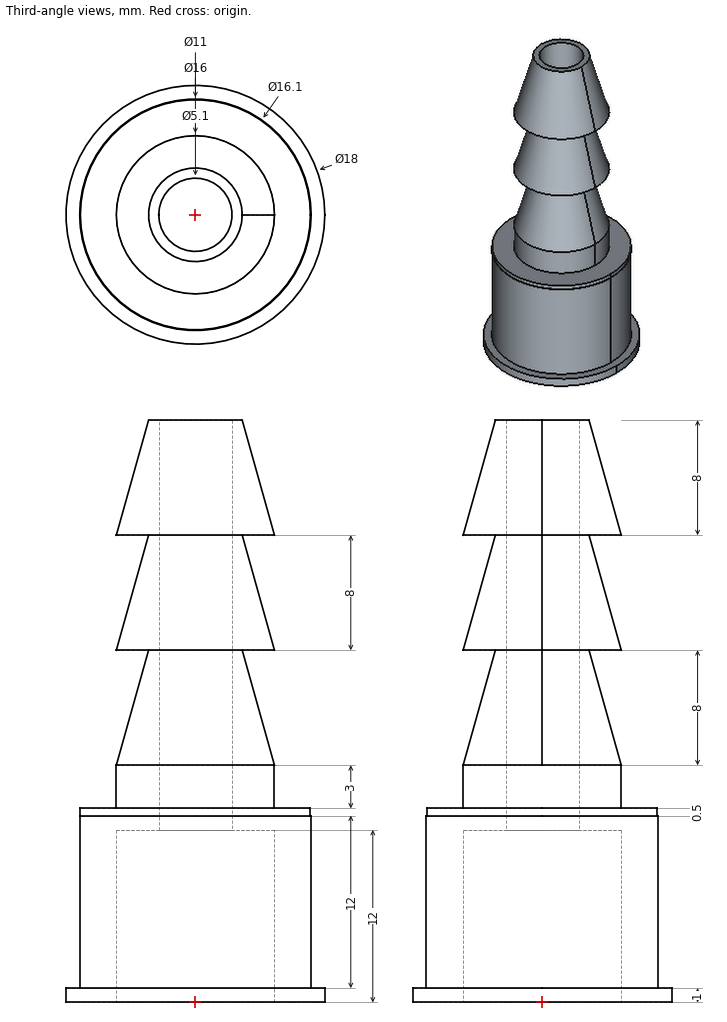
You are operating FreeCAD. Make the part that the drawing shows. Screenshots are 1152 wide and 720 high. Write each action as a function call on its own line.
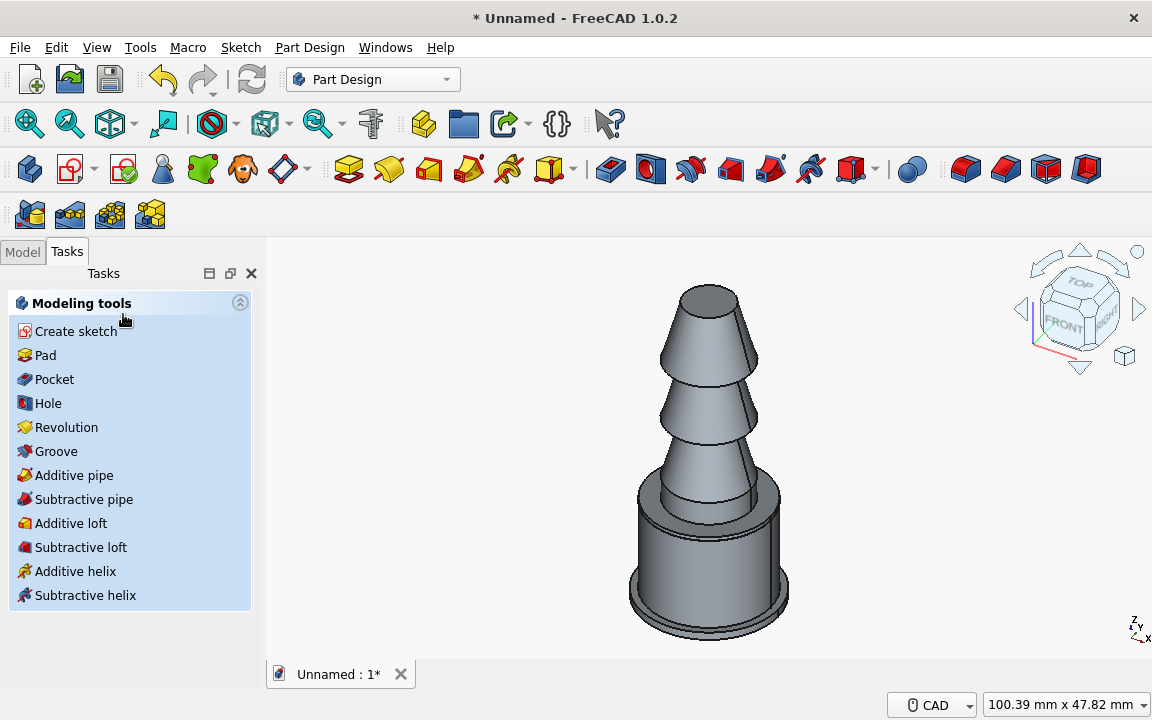
click(612, 170)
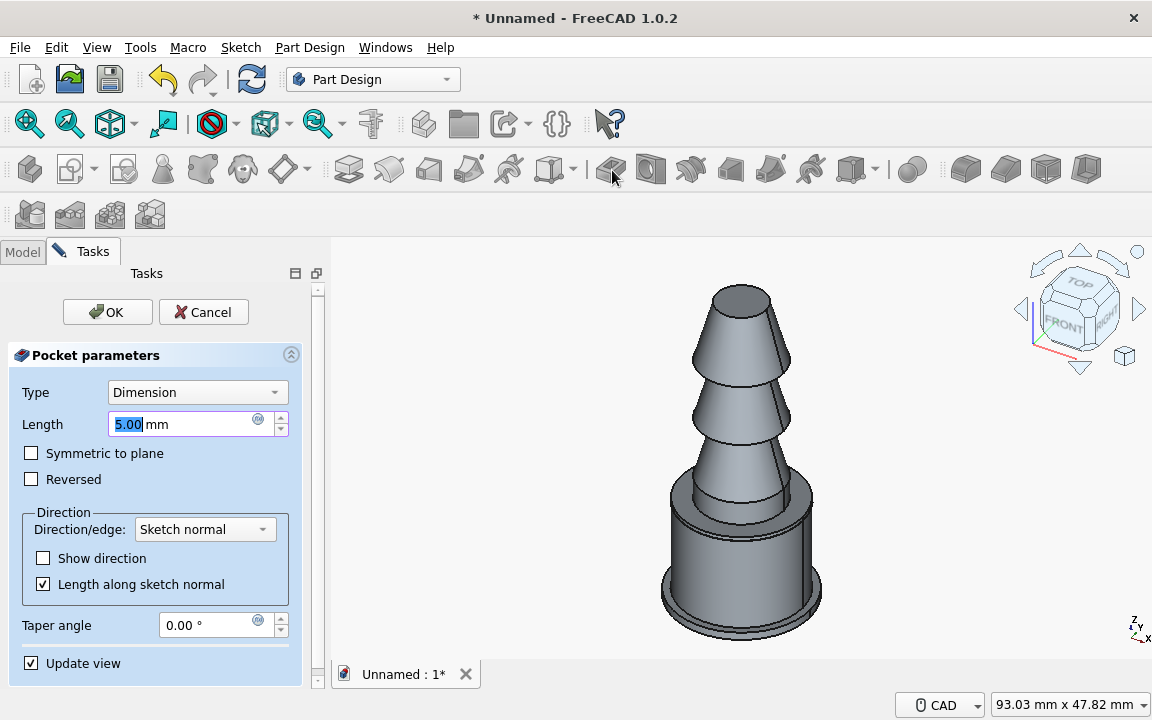
text(12)
key(Tab)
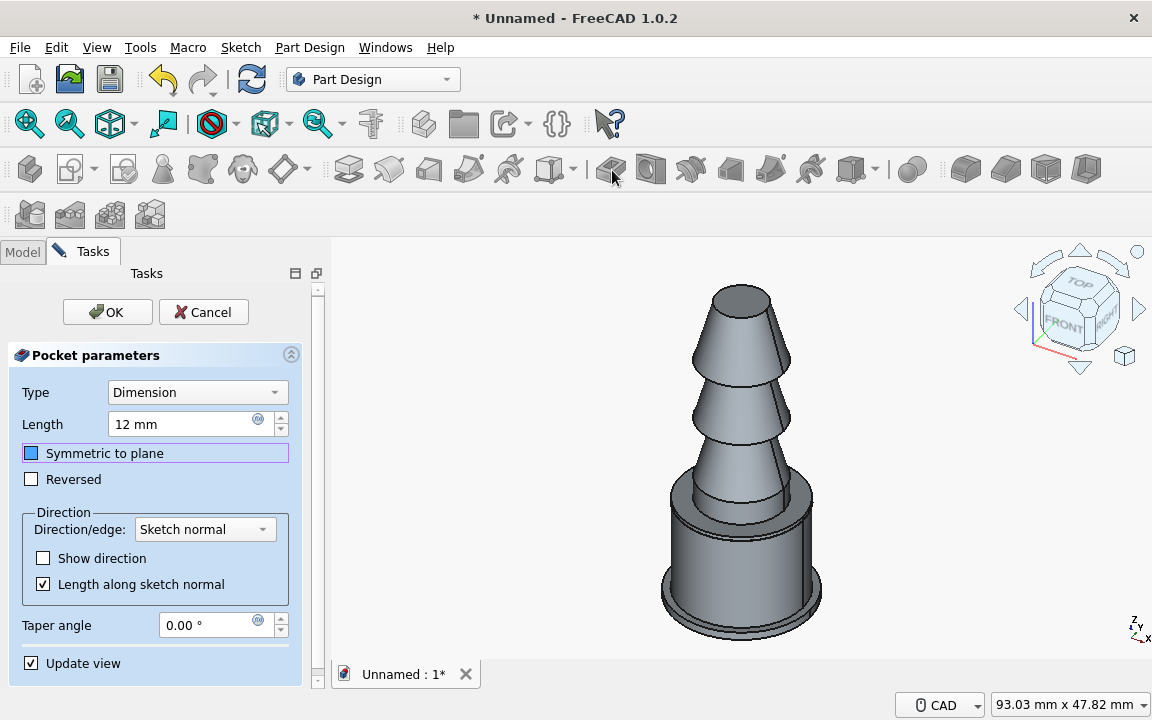
click(30, 479)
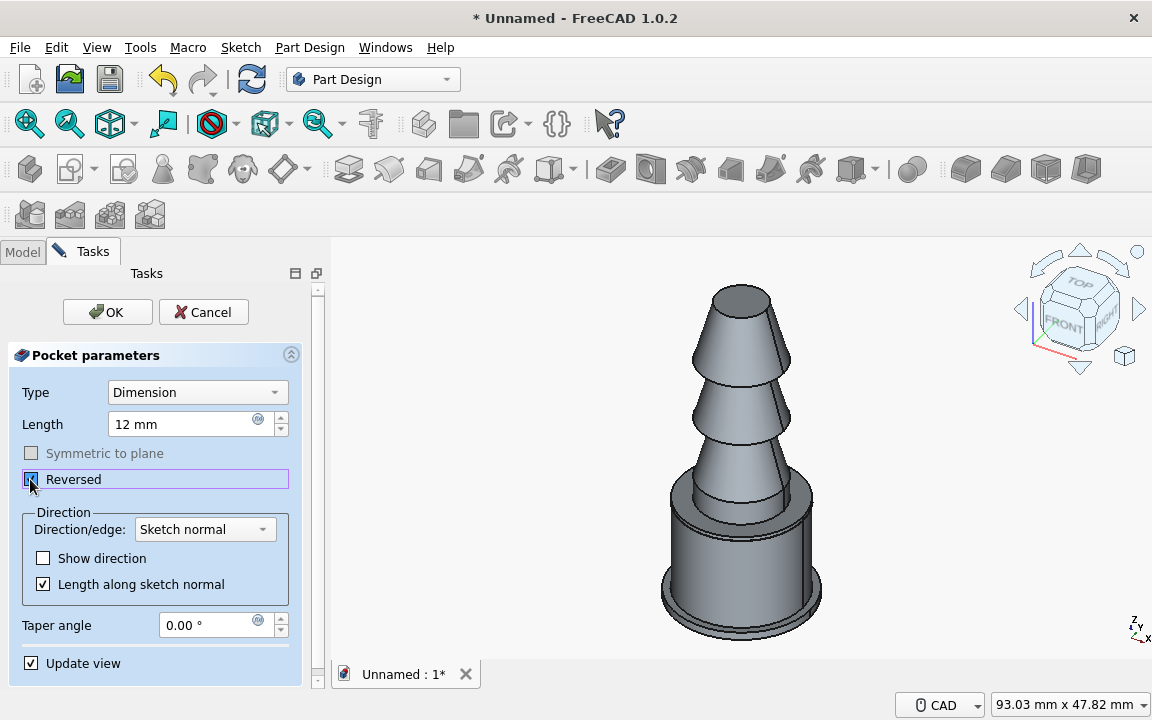
click(108, 312)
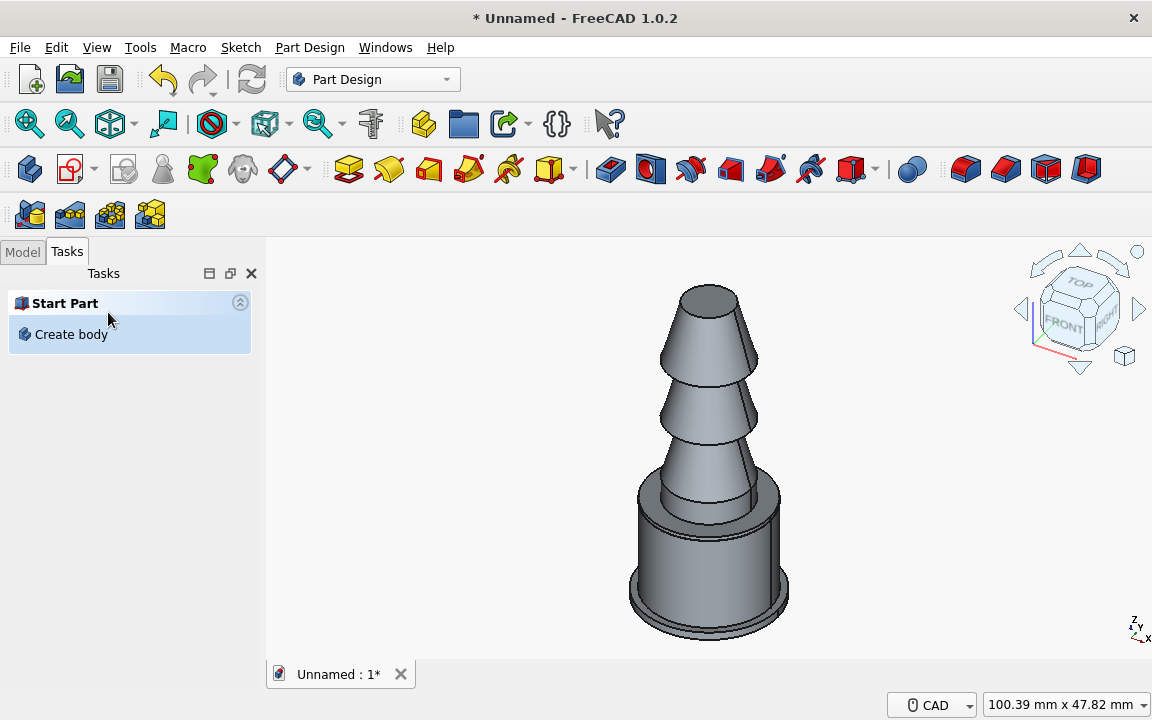
key(5)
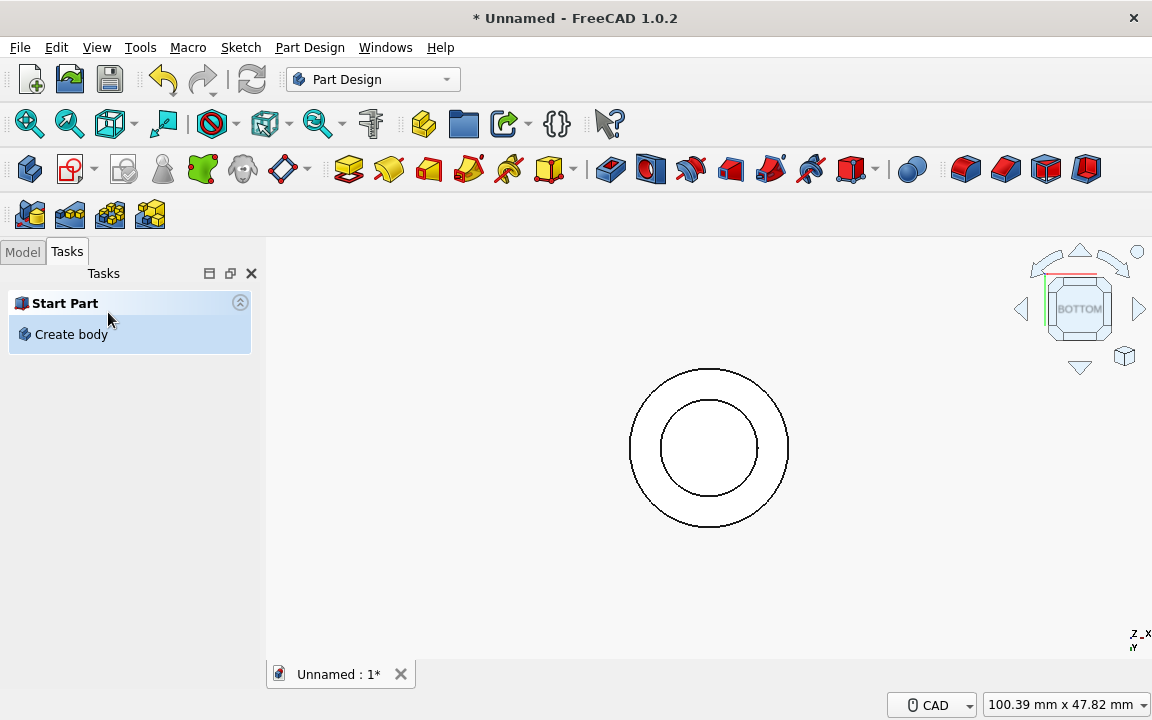
click(30, 124)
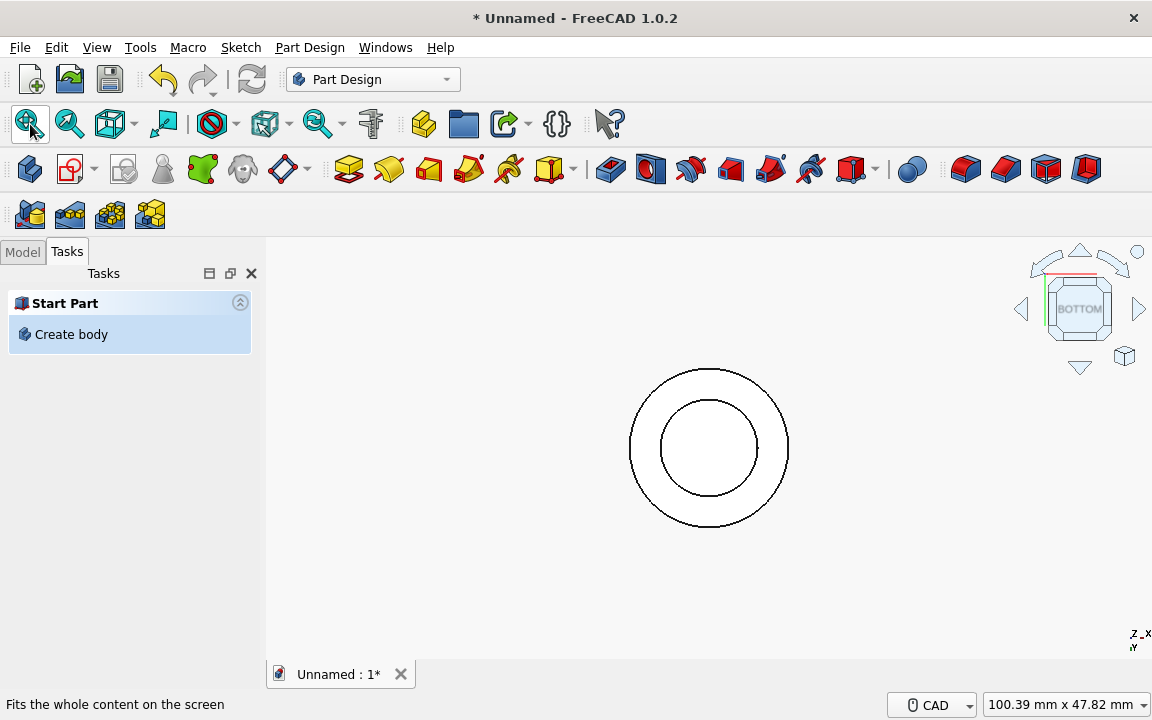
click(709, 447)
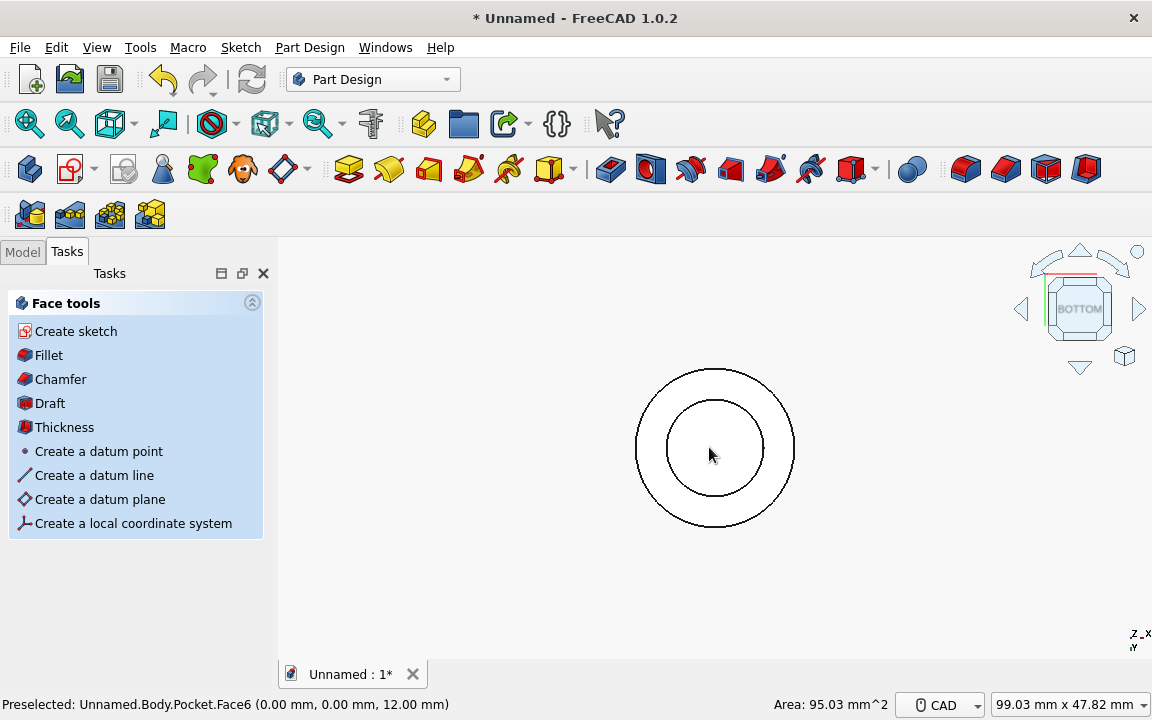
click(70, 170)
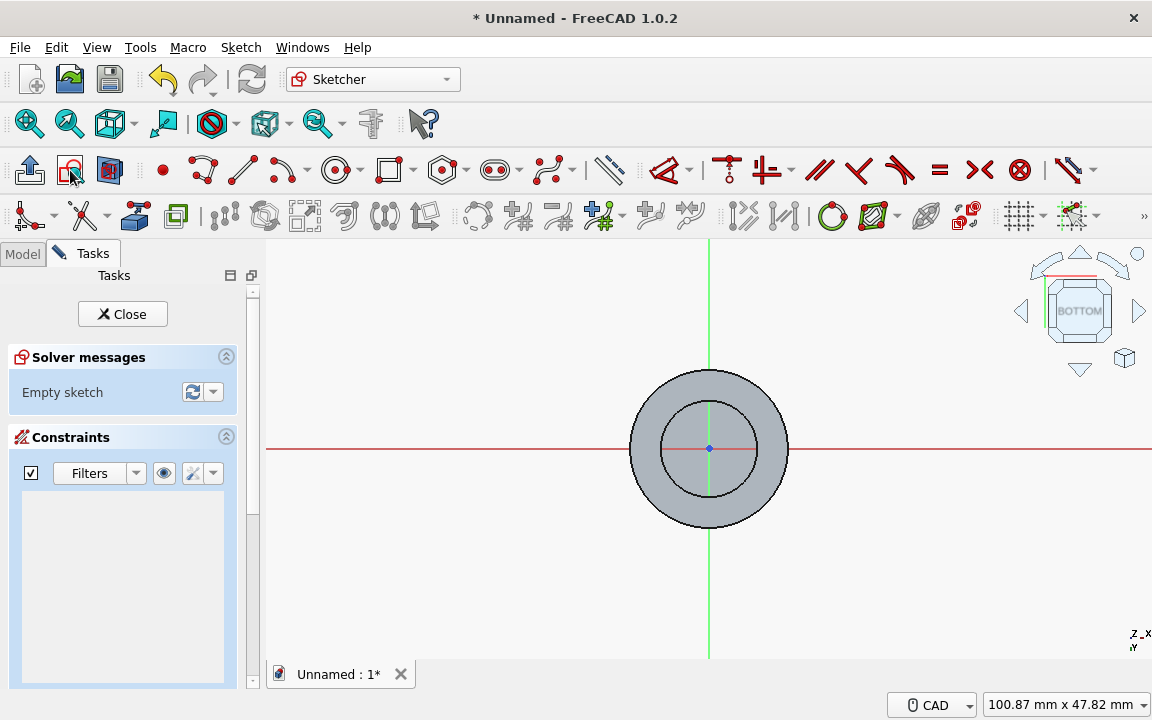
scroll(723, 449, up, 9)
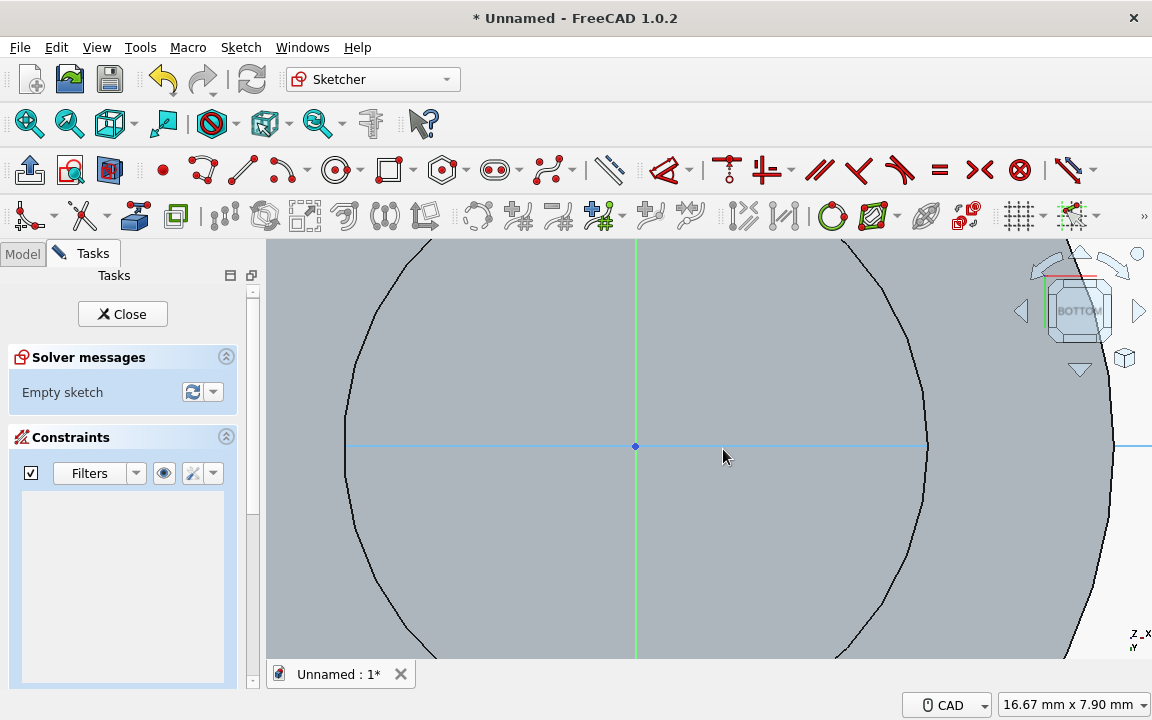
click(336, 170)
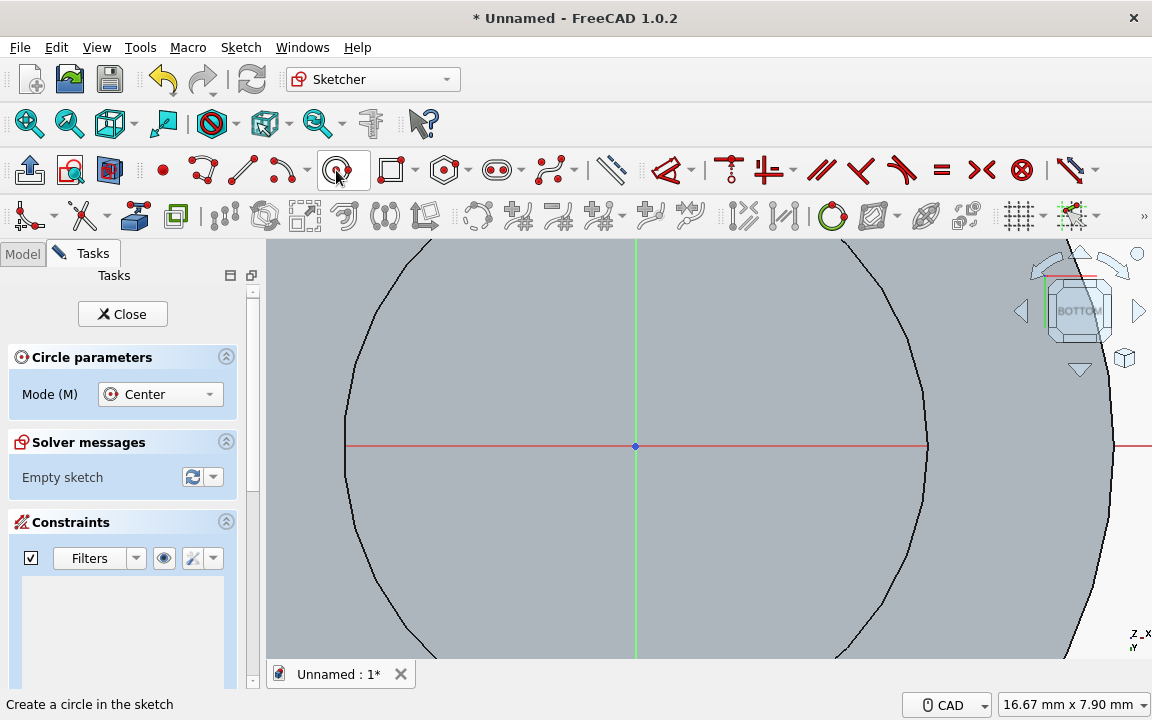
click(636, 446)
click(732, 351)
key(Escape)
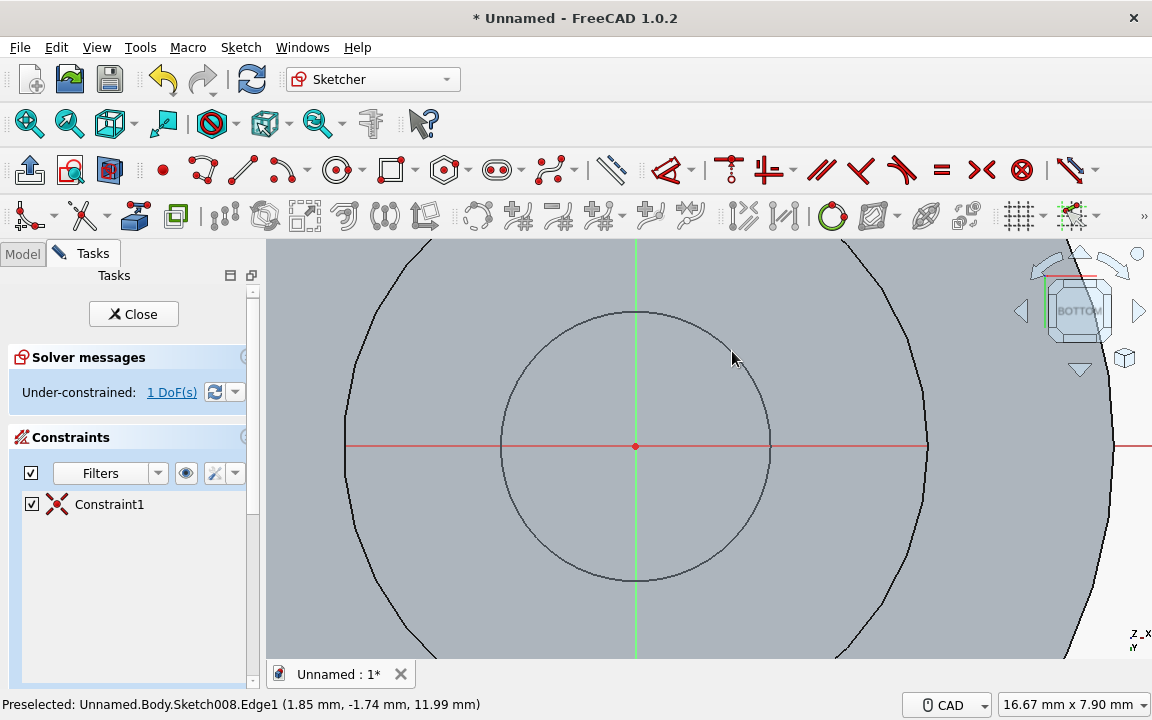
key(d)